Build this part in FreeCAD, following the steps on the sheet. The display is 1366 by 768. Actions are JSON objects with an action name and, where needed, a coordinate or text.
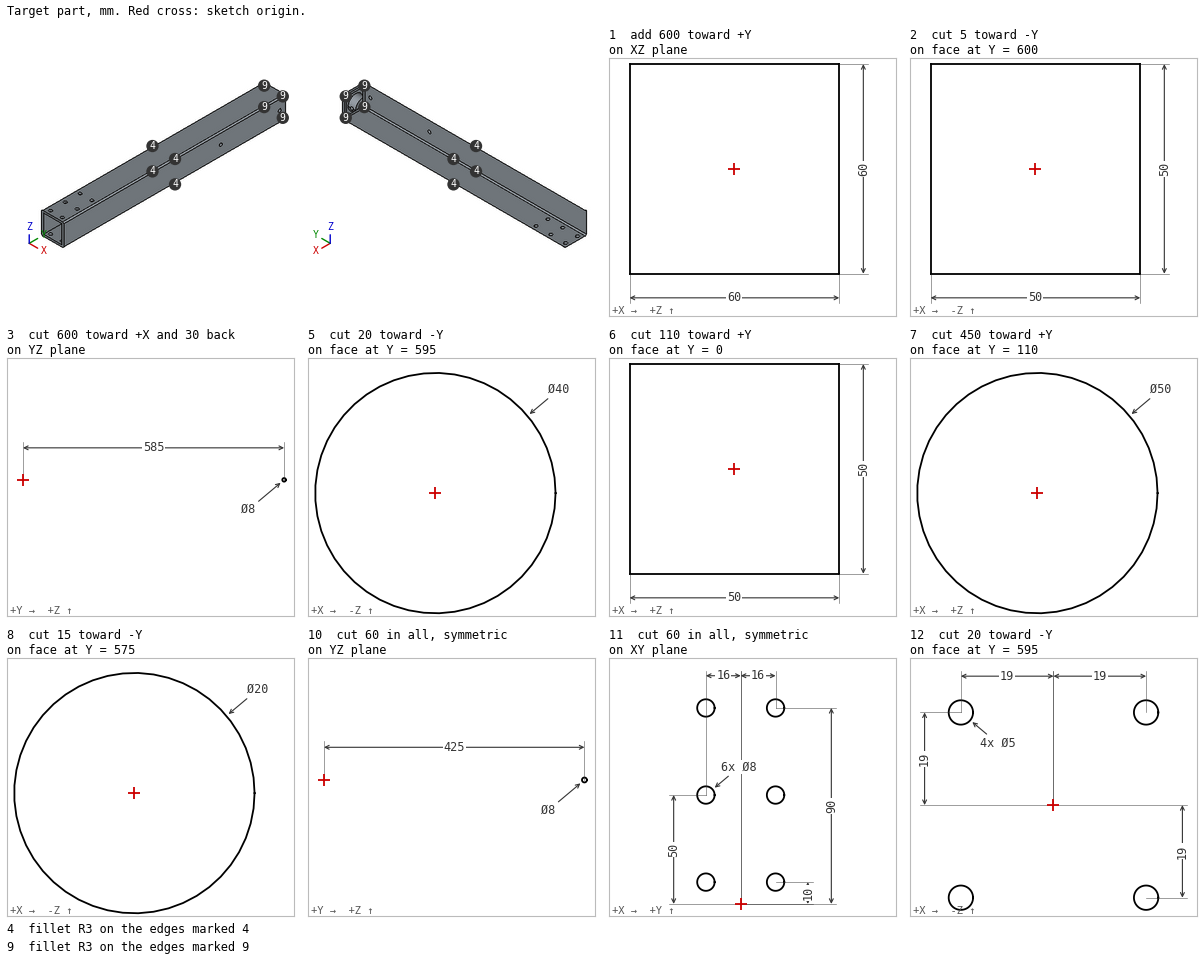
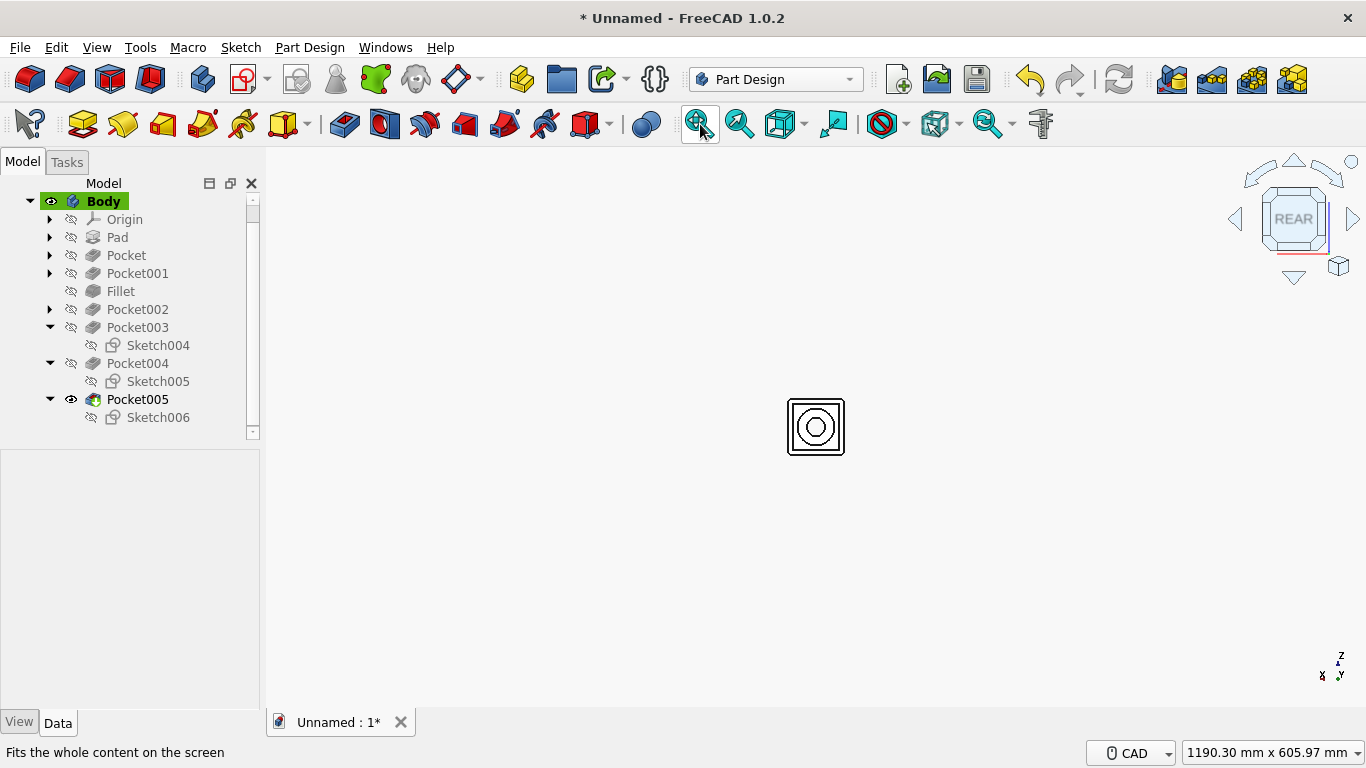
{"action": "key", "text": "6"}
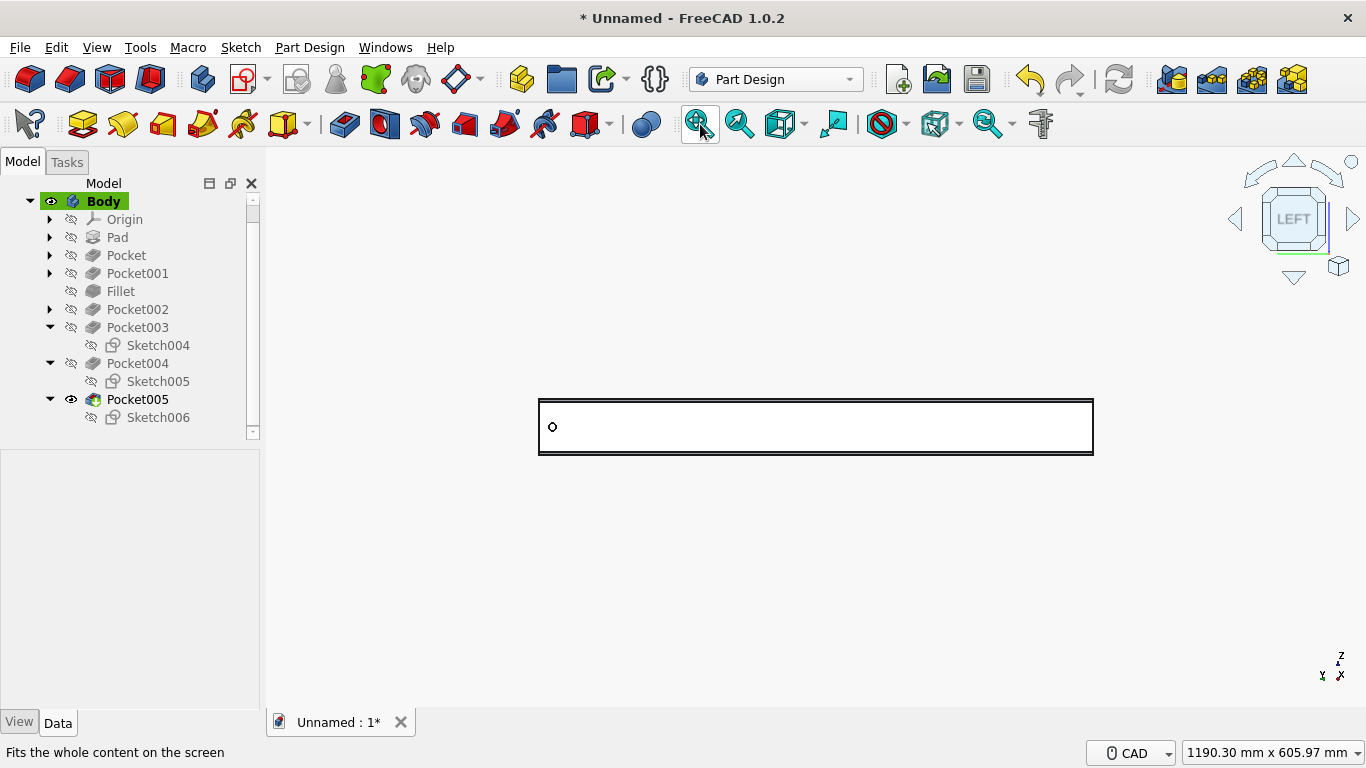
{"action": "scroll", "coordinate": [541, 449], "scroll_direction": "up", "scroll_amount": 11}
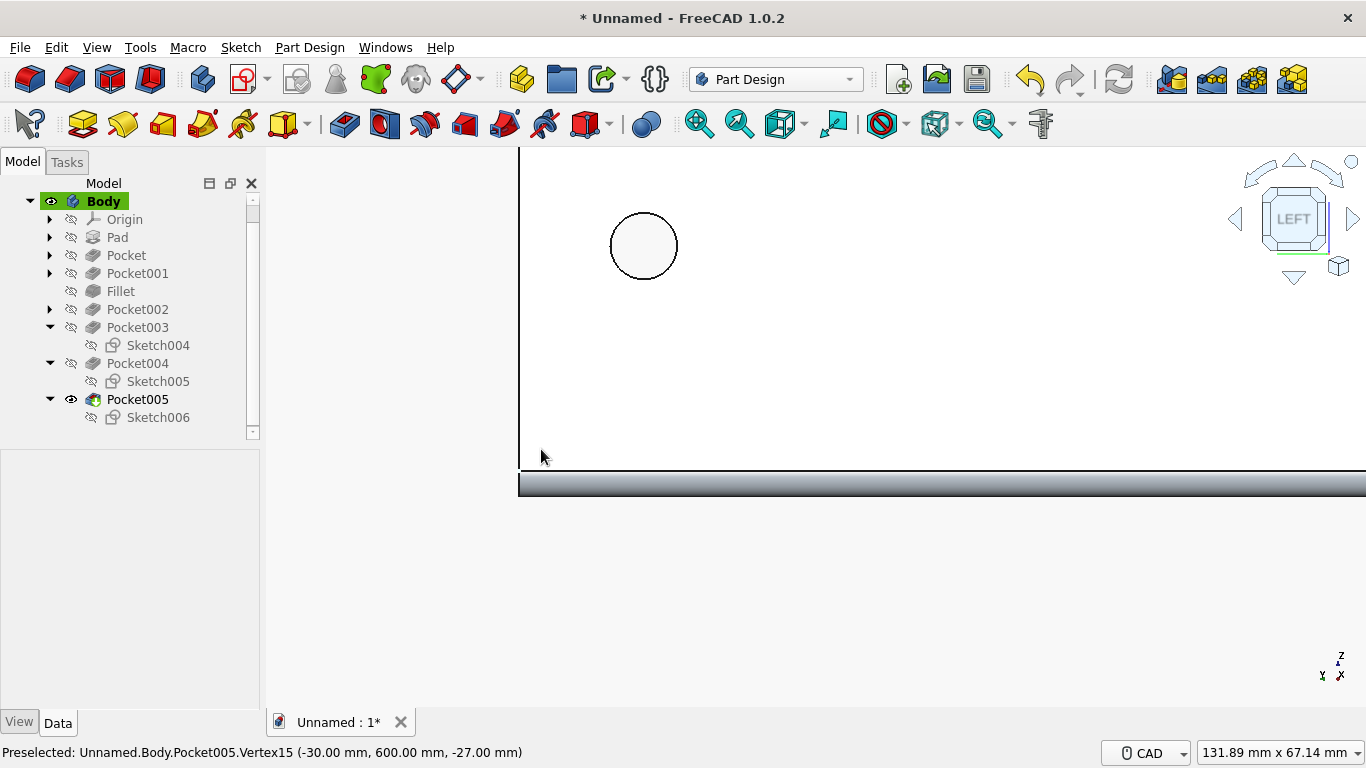
{"action": "left_click", "coordinate": [700, 124]}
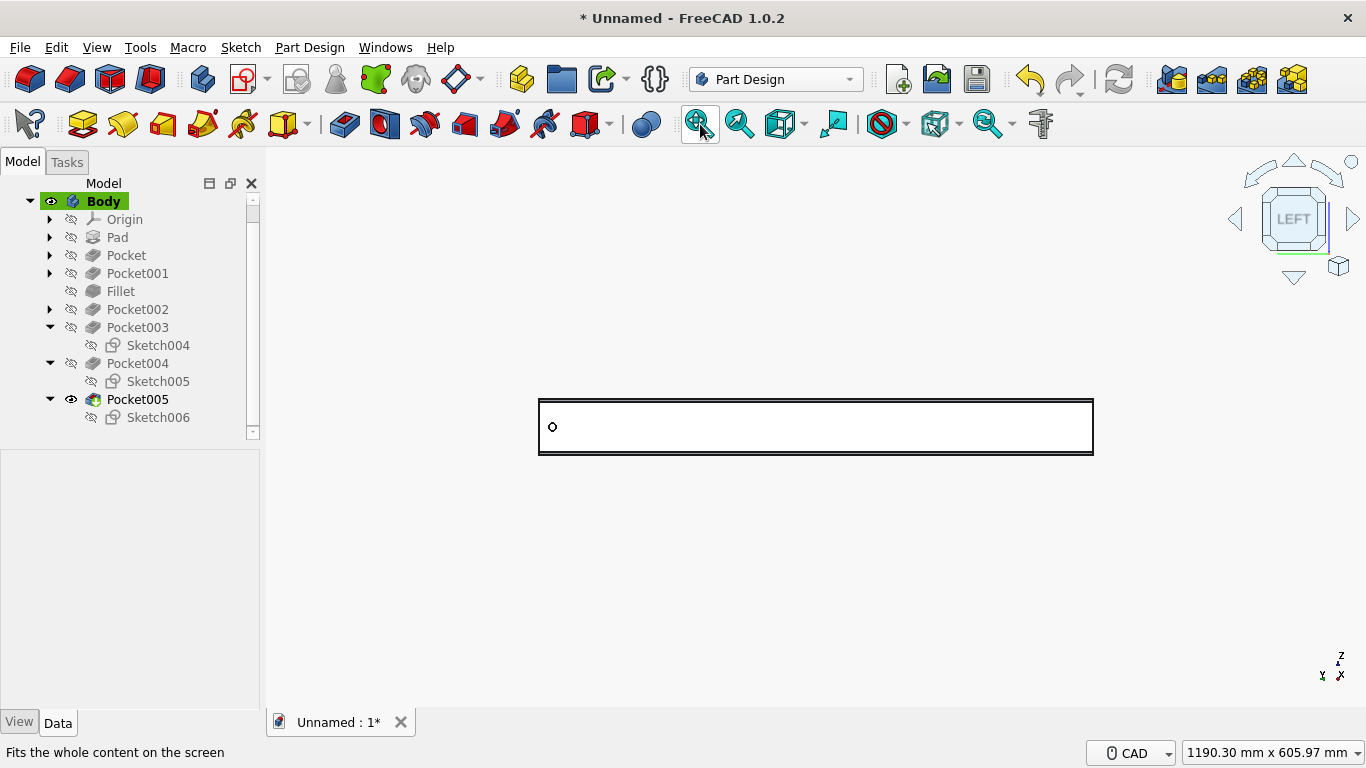
{"action": "key", "text": "v 3"}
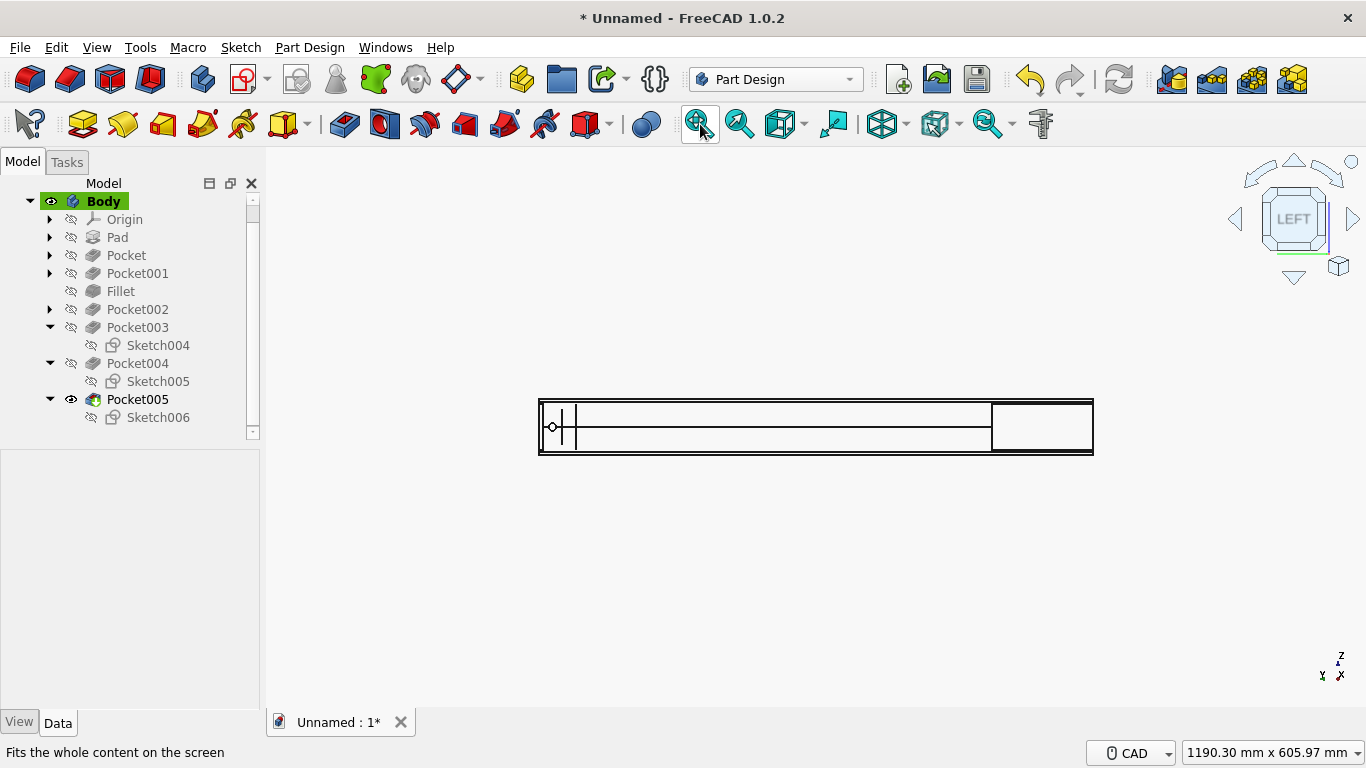
{"action": "key", "text": "0"}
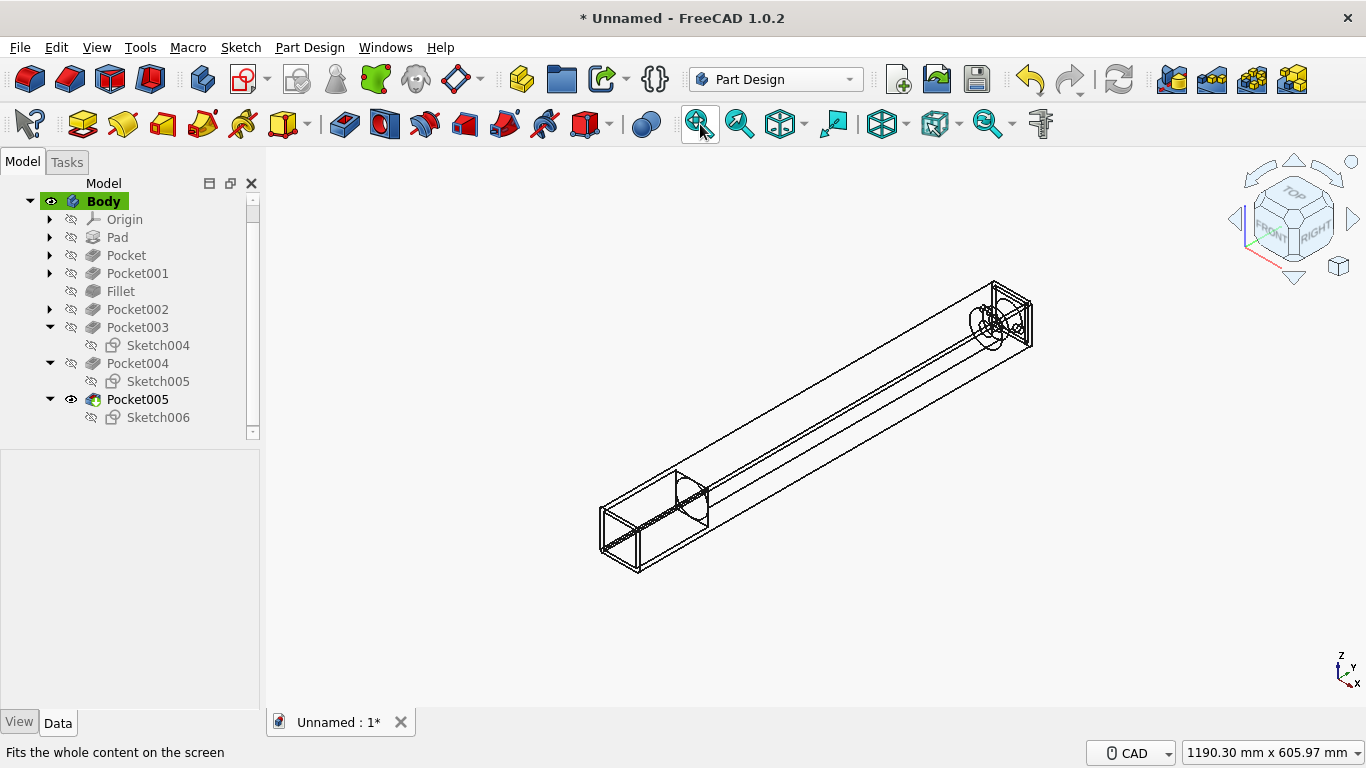
{"action": "scroll", "coordinate": [1027, 342], "scroll_direction": "up", "scroll_amount": 11}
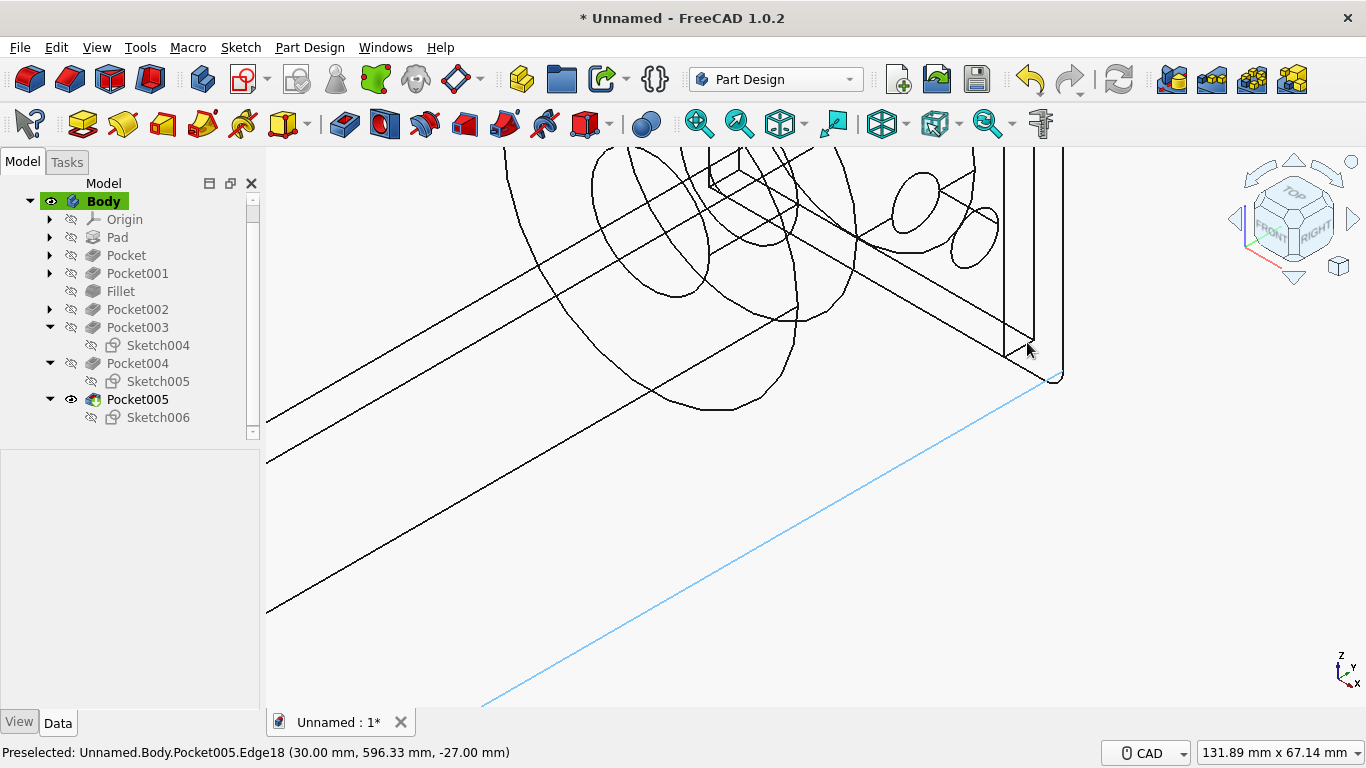
{"action": "left_click", "coordinate": [1019, 348]}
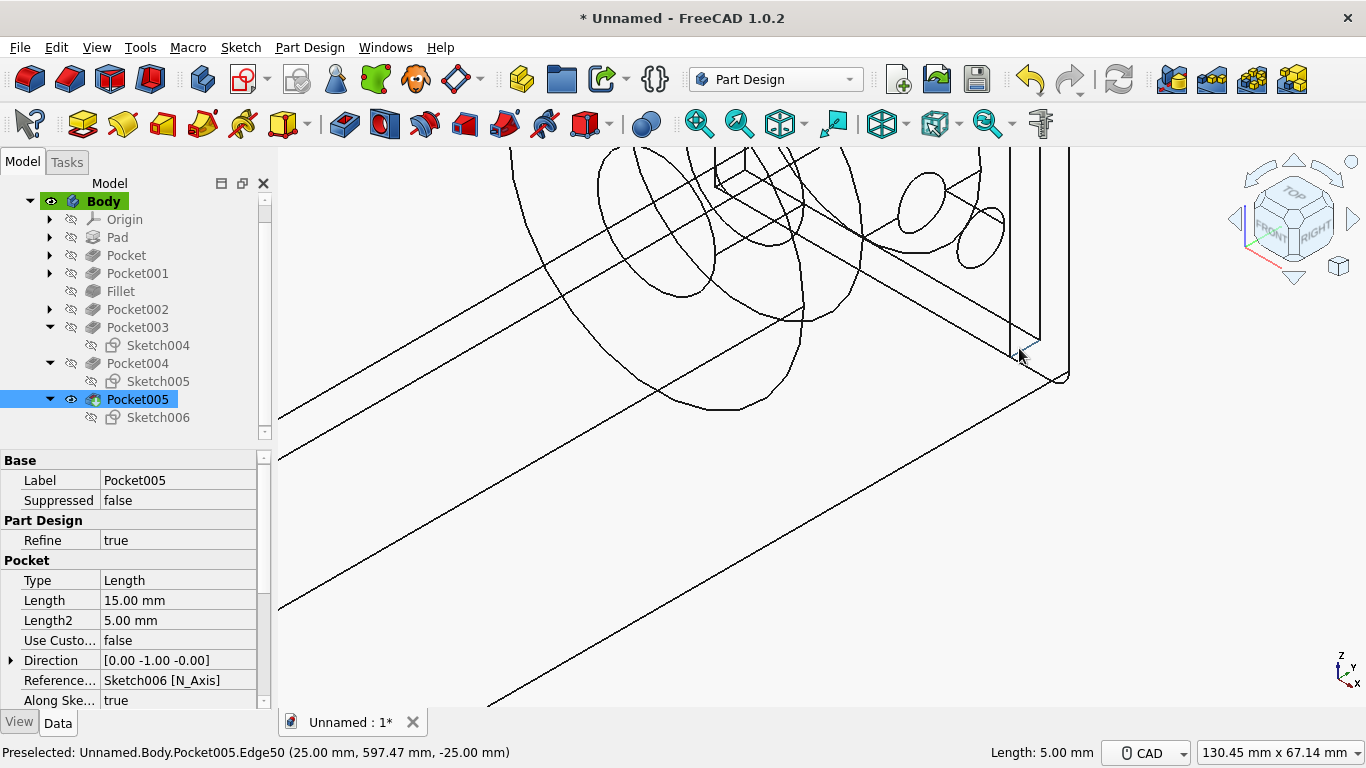
{"action": "left_click", "coordinate": [730, 177], "text": "ctrl"}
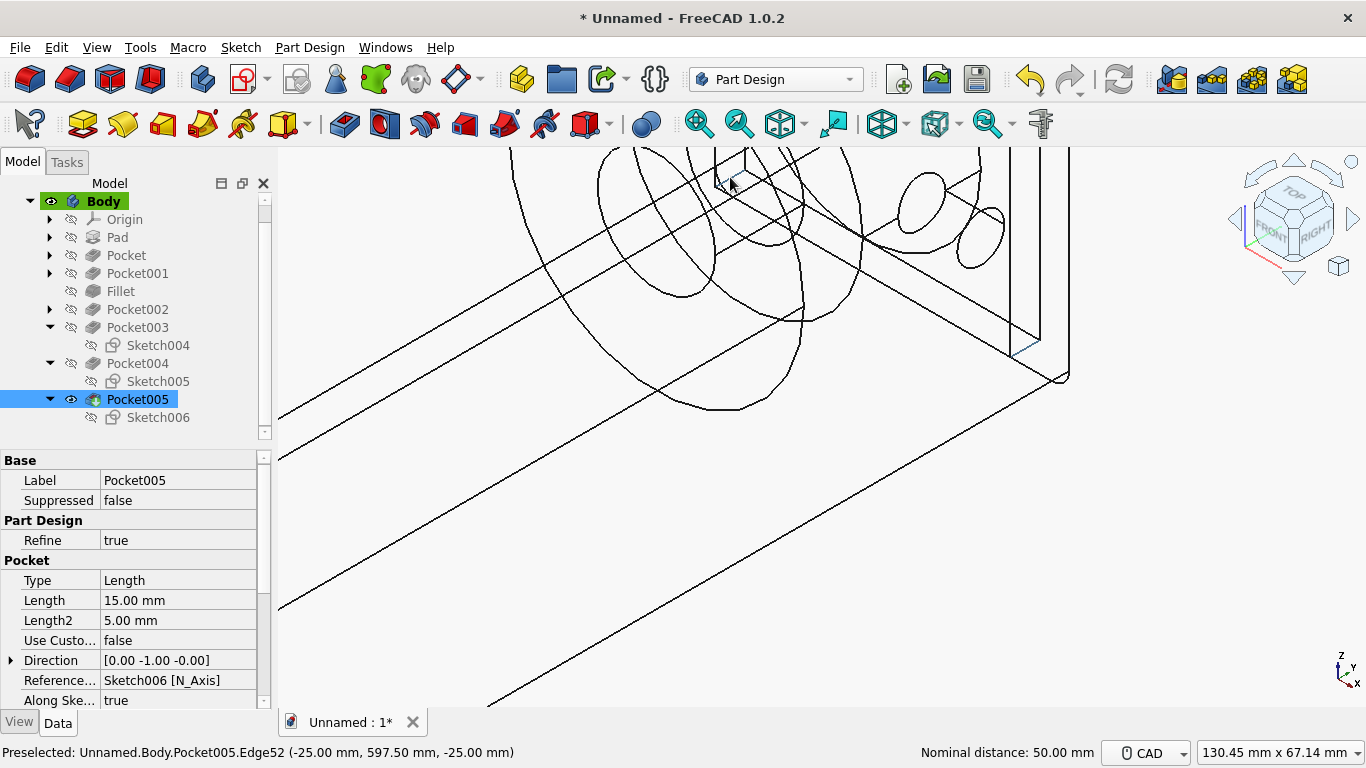
{"action": "key", "text": "v f"}